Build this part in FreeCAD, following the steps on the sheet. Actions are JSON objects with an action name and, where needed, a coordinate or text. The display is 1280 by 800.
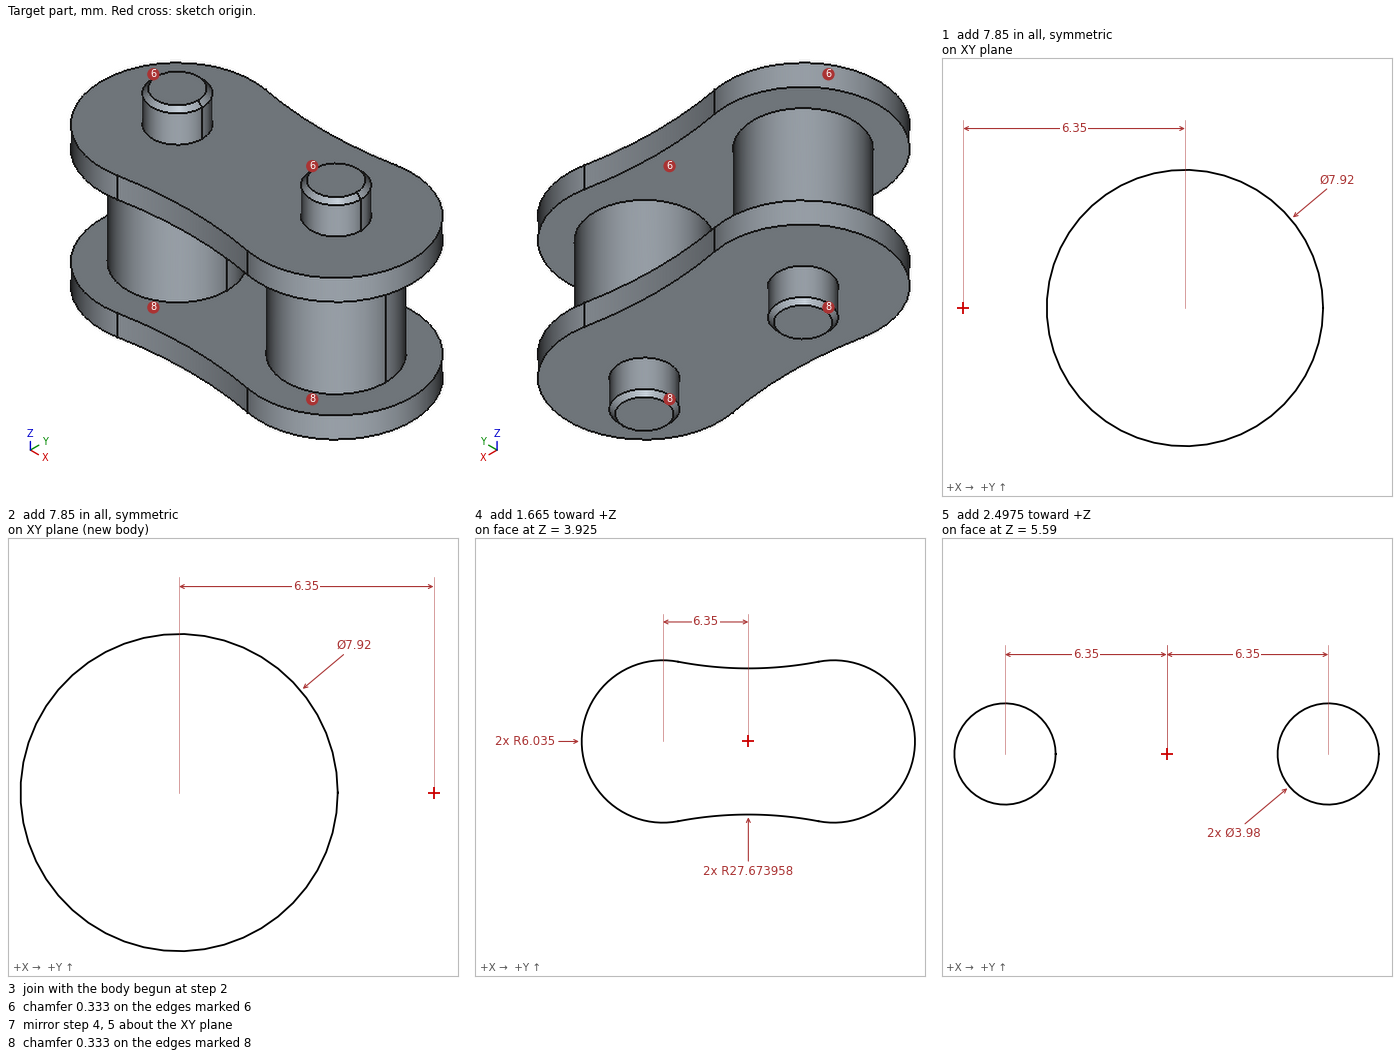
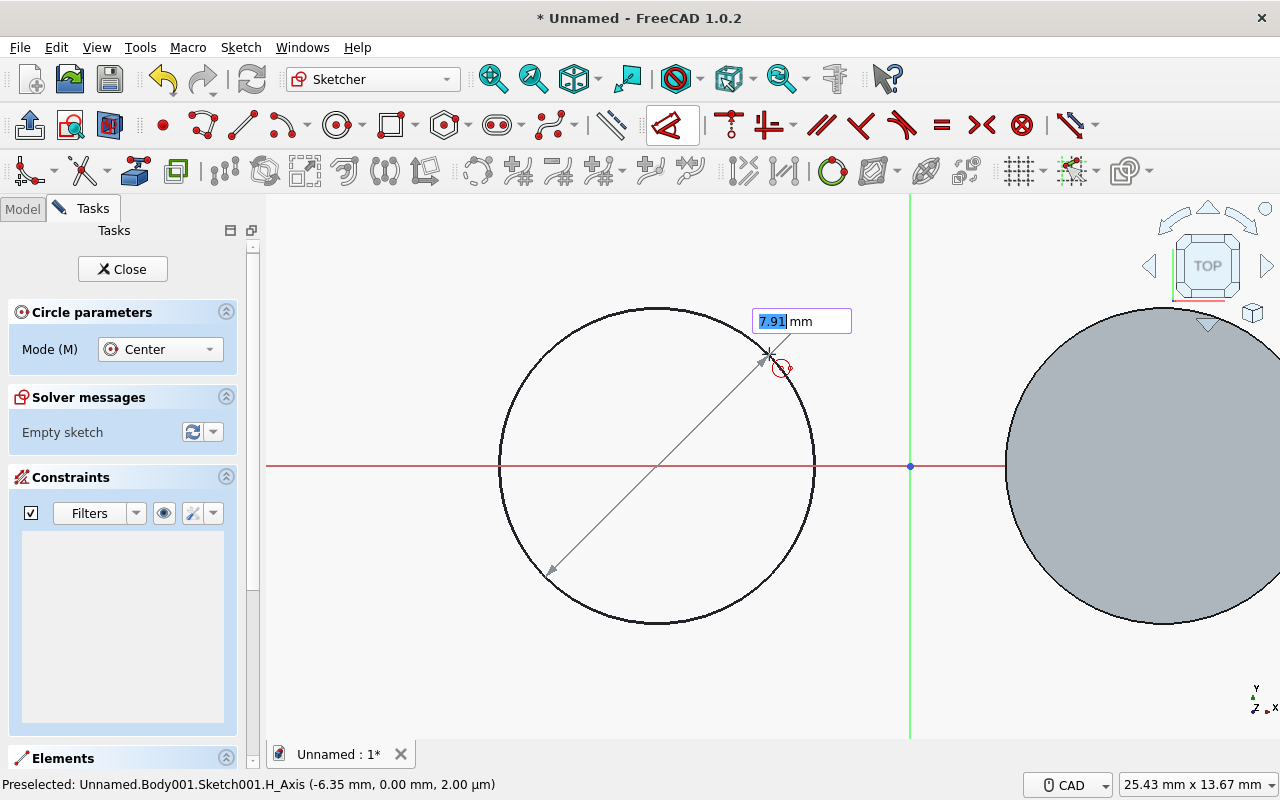
{"action": "type", "text": "7.92"}
{"action": "key", "text": "Return"}
{"action": "key", "text": "Escape"}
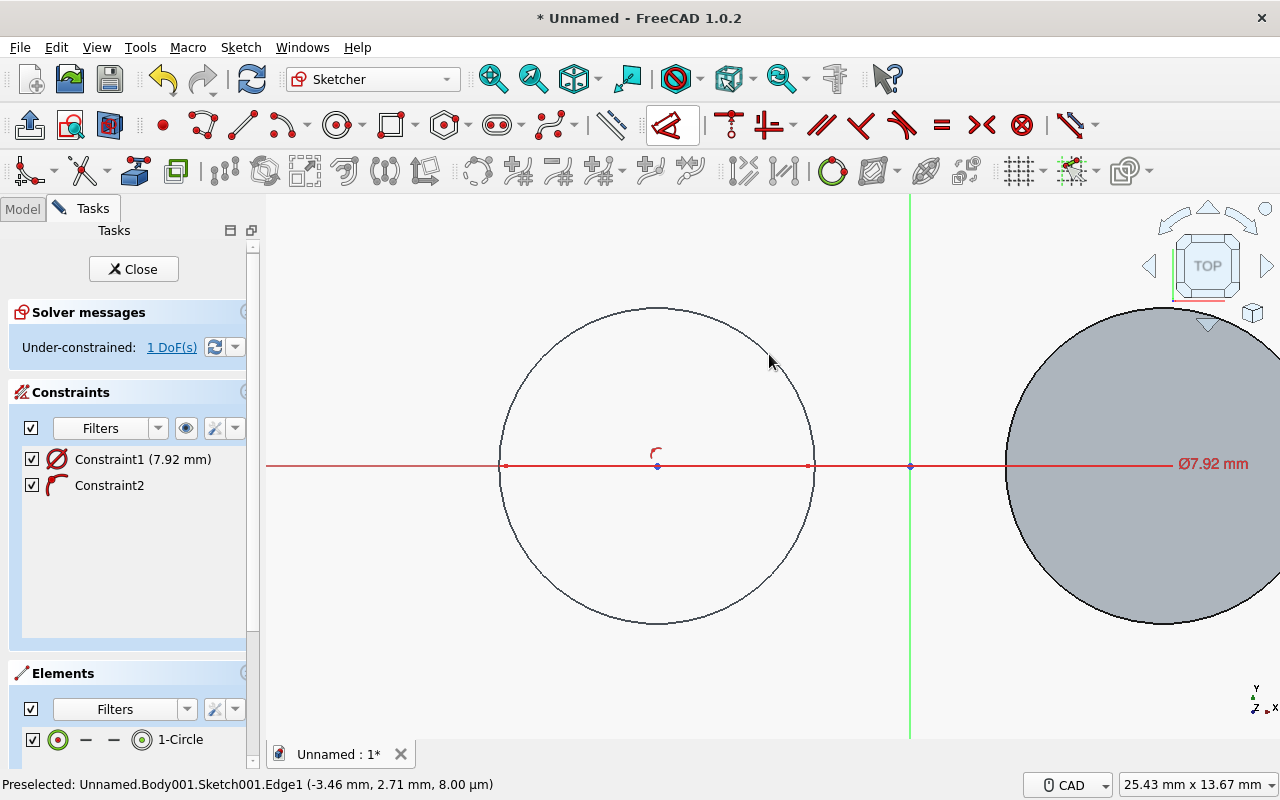
{"action": "left_click", "coordinate": [657, 466]}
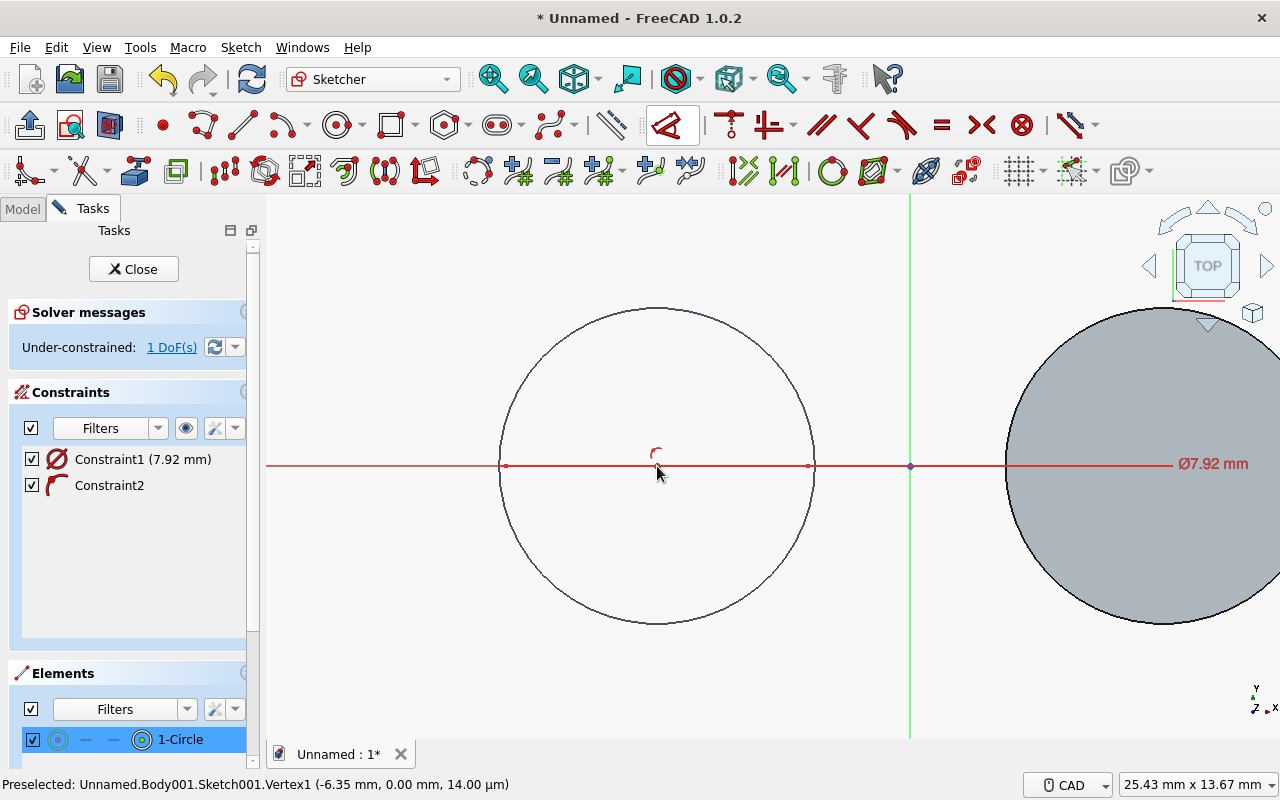
{"action": "key", "text": "l"}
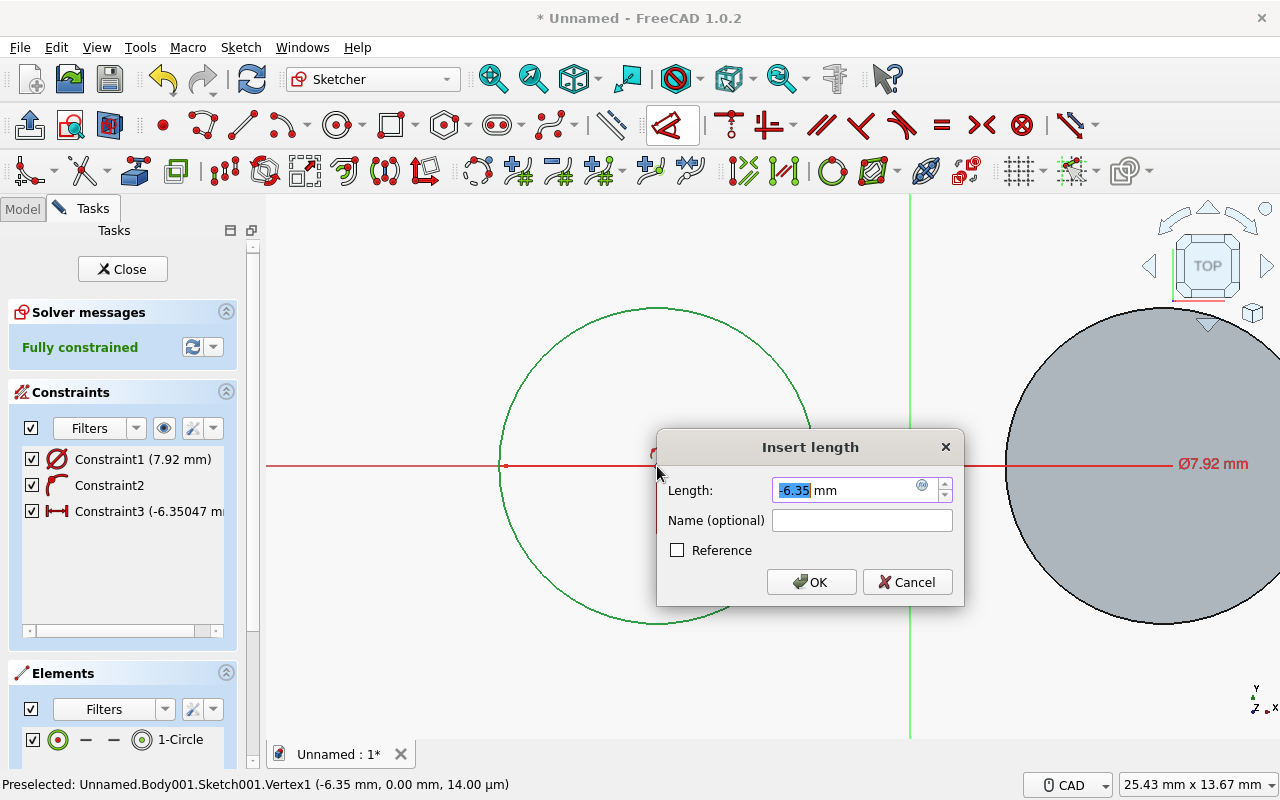
{"action": "type", "text": "-6.35"}
{"action": "key", "text": "Return"}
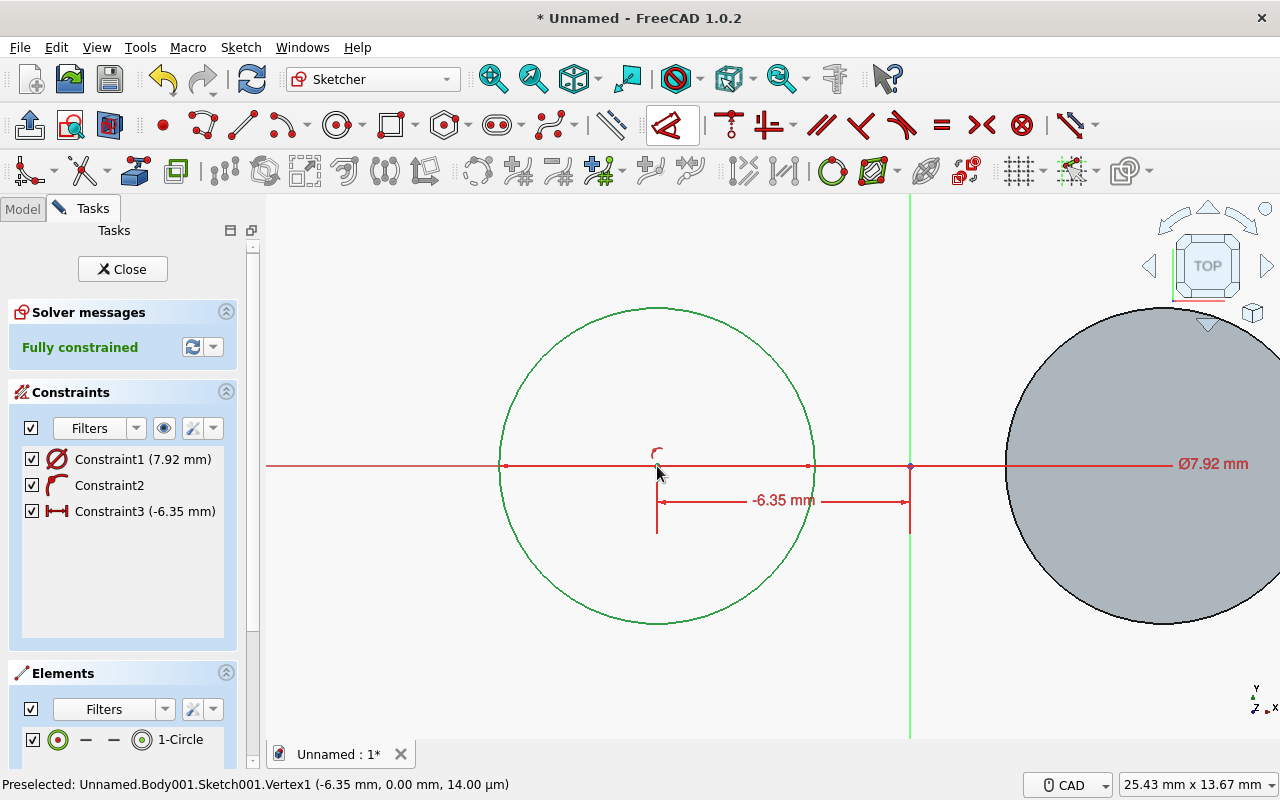
{"action": "left_click", "coordinate": [123, 269]}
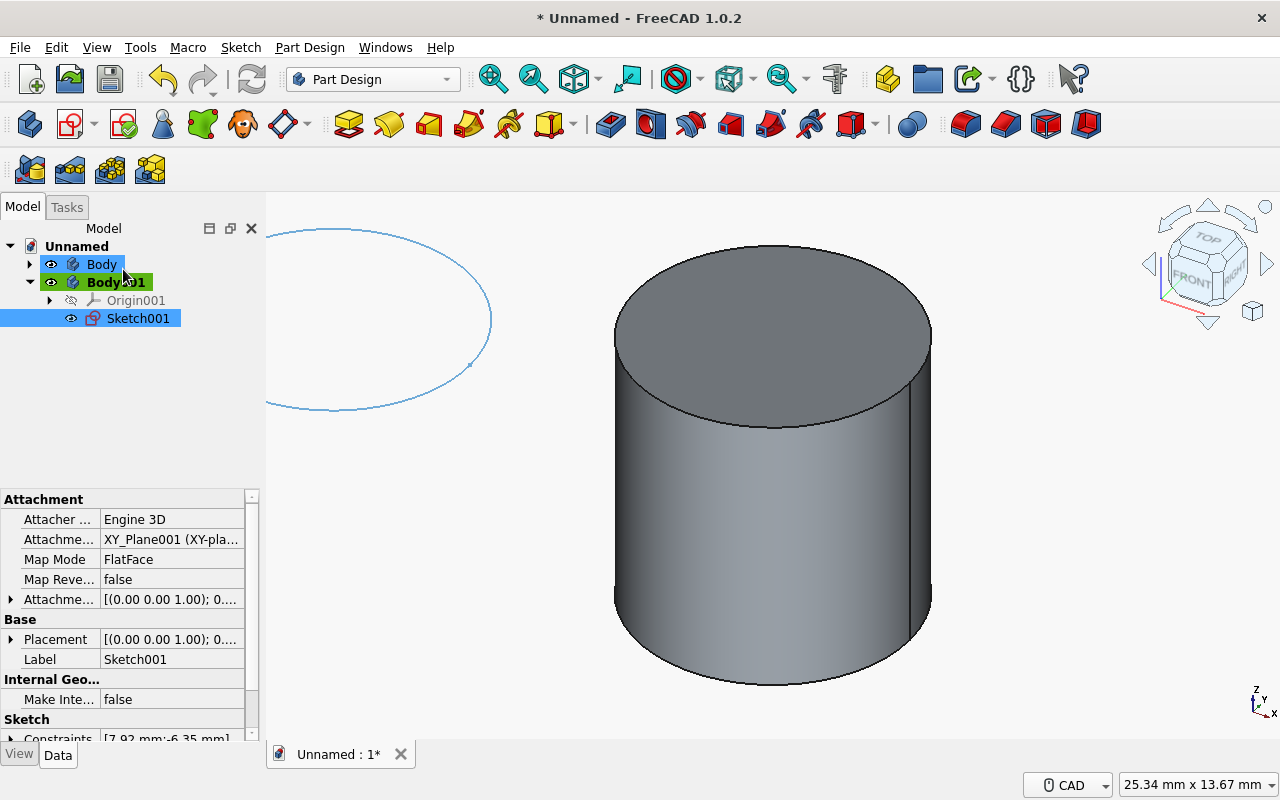
{"action": "left_click", "coordinate": [350, 124]}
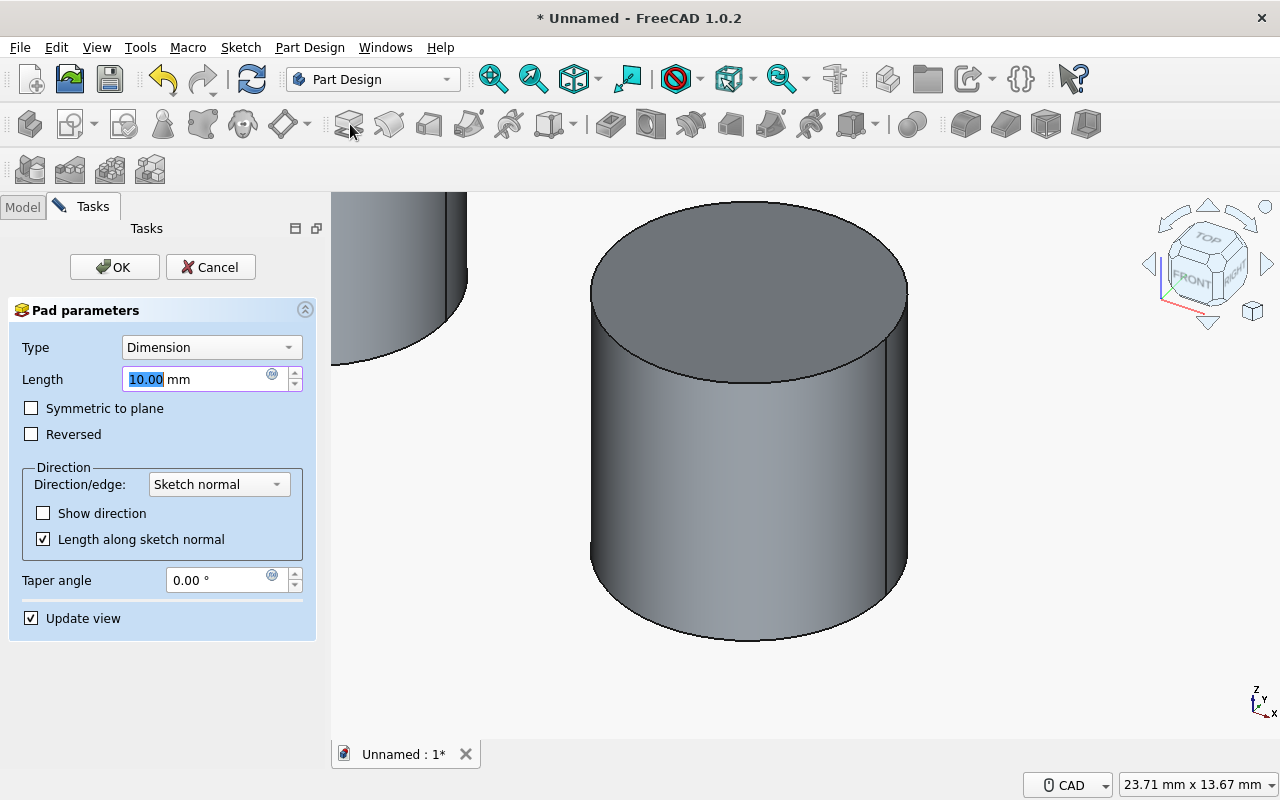
{"action": "type", "text": "7.85"}
{"action": "key", "text": "Tab"}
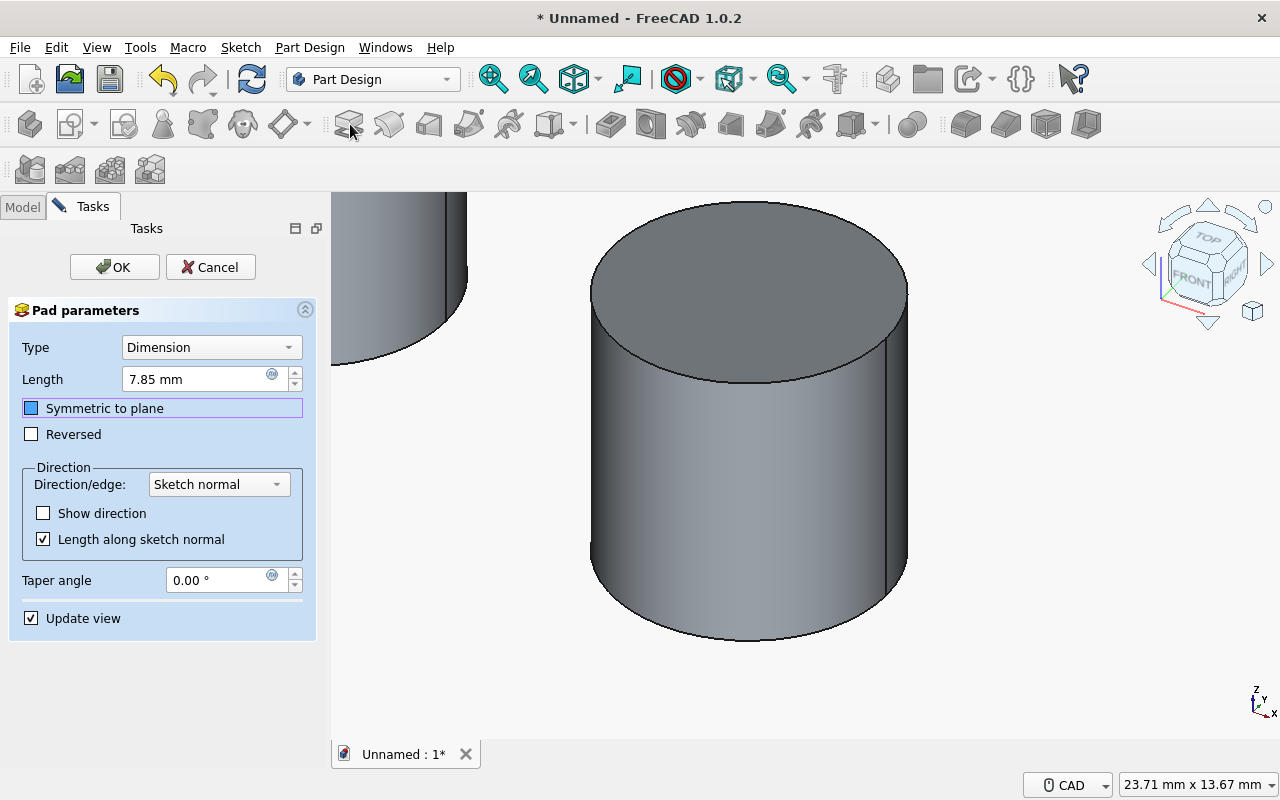
{"action": "left_click", "coordinate": [30, 408]}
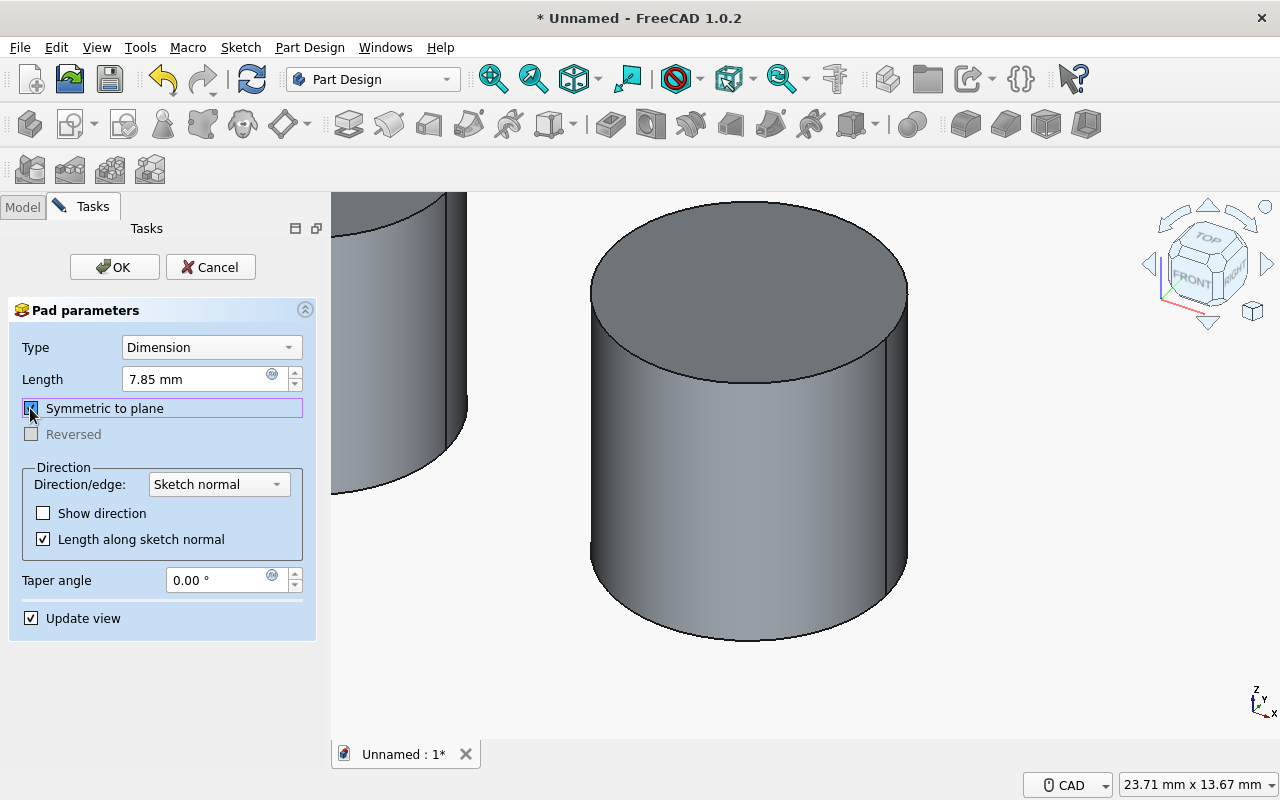
{"action": "left_click", "coordinate": [115, 267]}